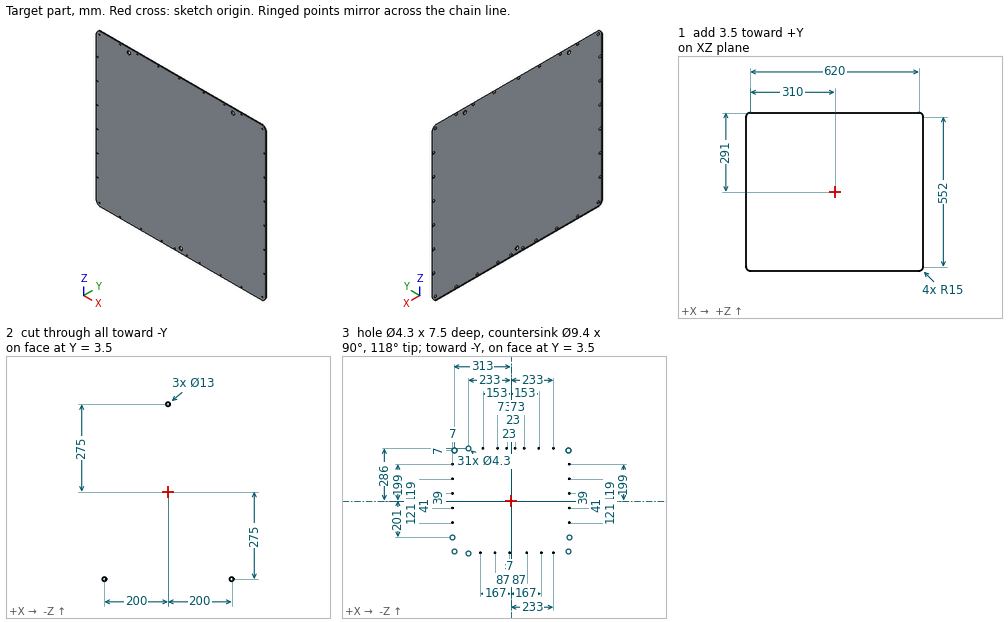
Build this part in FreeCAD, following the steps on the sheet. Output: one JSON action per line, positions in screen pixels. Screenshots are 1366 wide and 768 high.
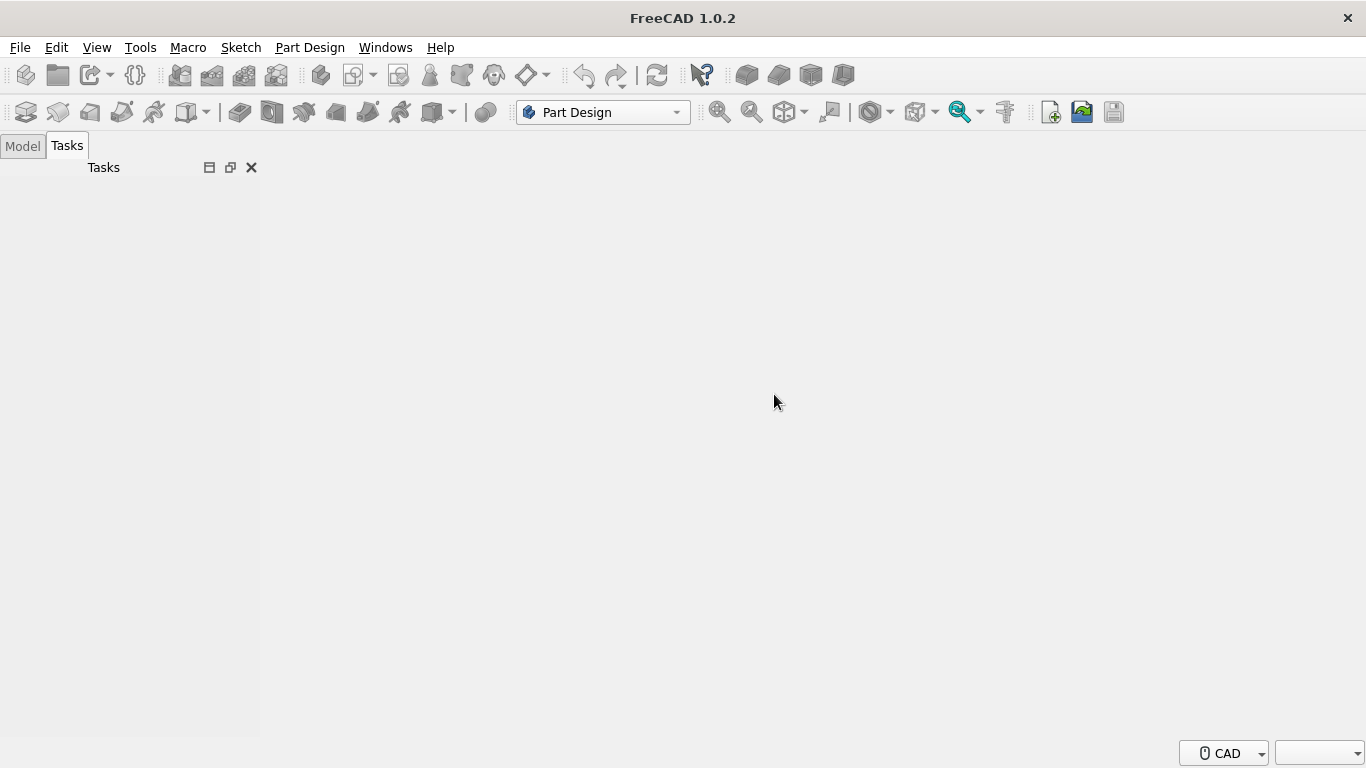
{"action": "left_click", "coordinate": [1050, 112]}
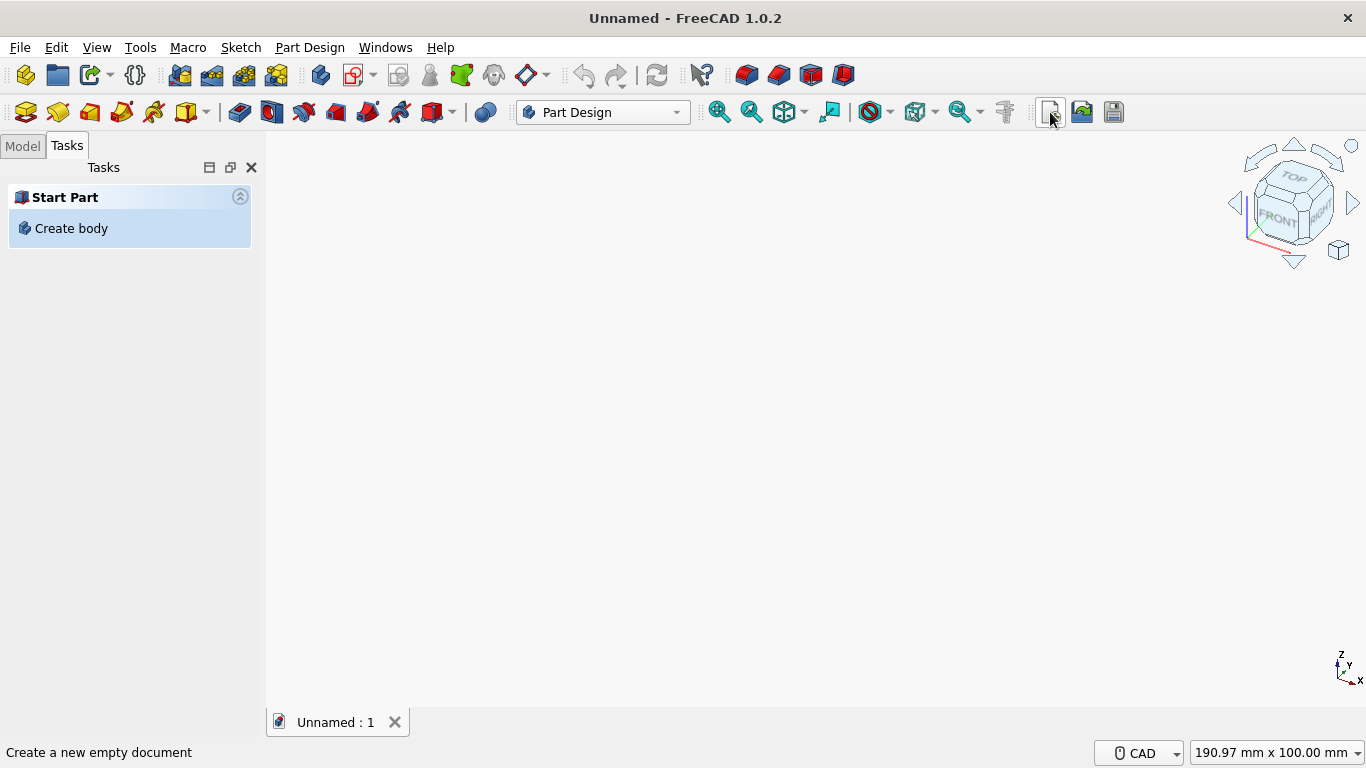
{"action": "left_click", "coordinate": [354, 76]}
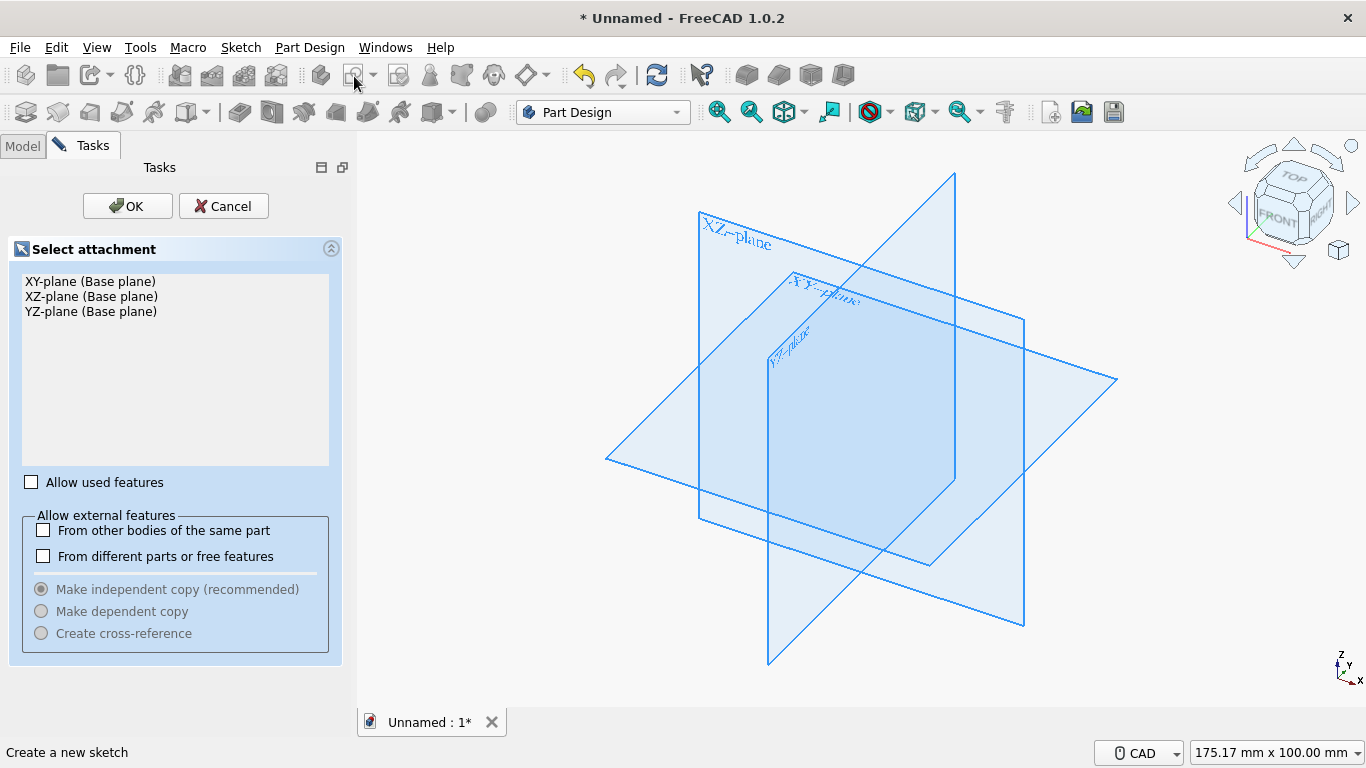
{"action": "left_click", "coordinate": [82, 296]}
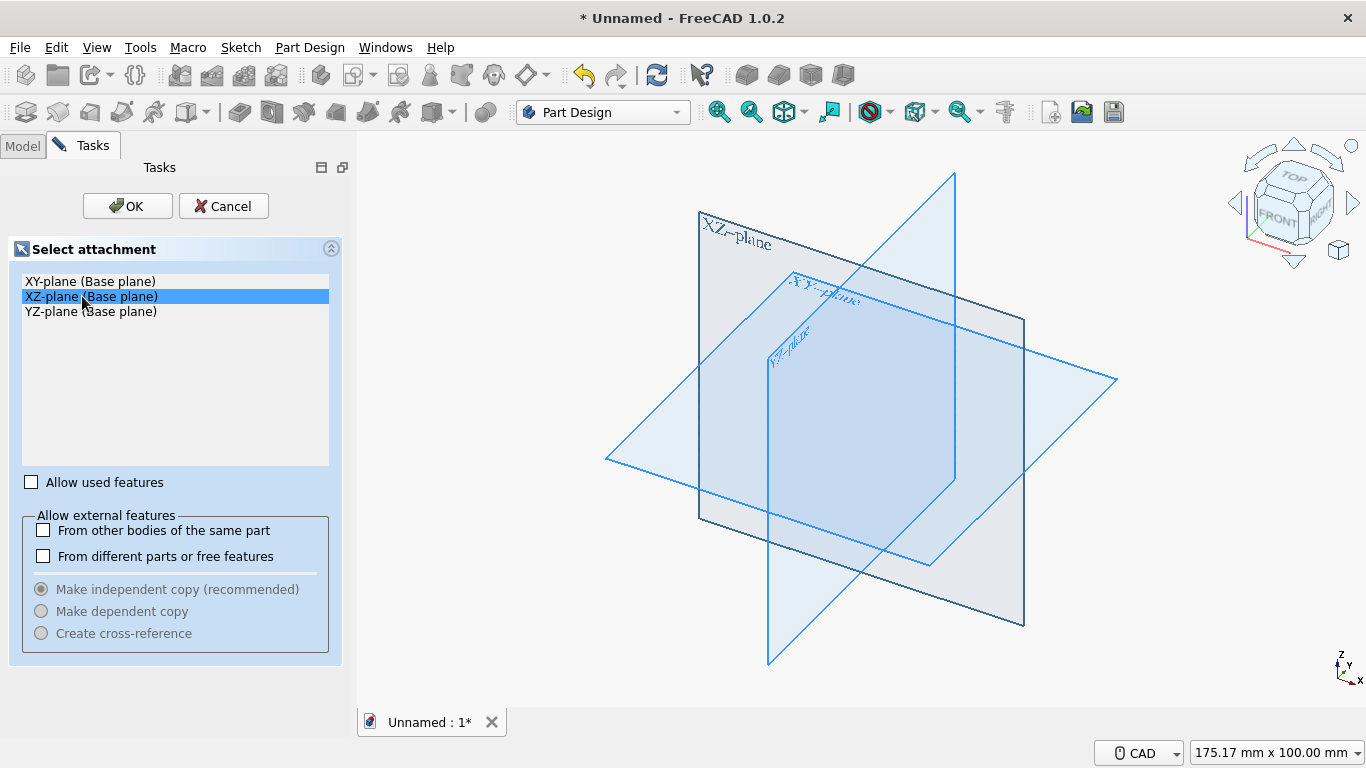
{"action": "left_click", "coordinate": [128, 206]}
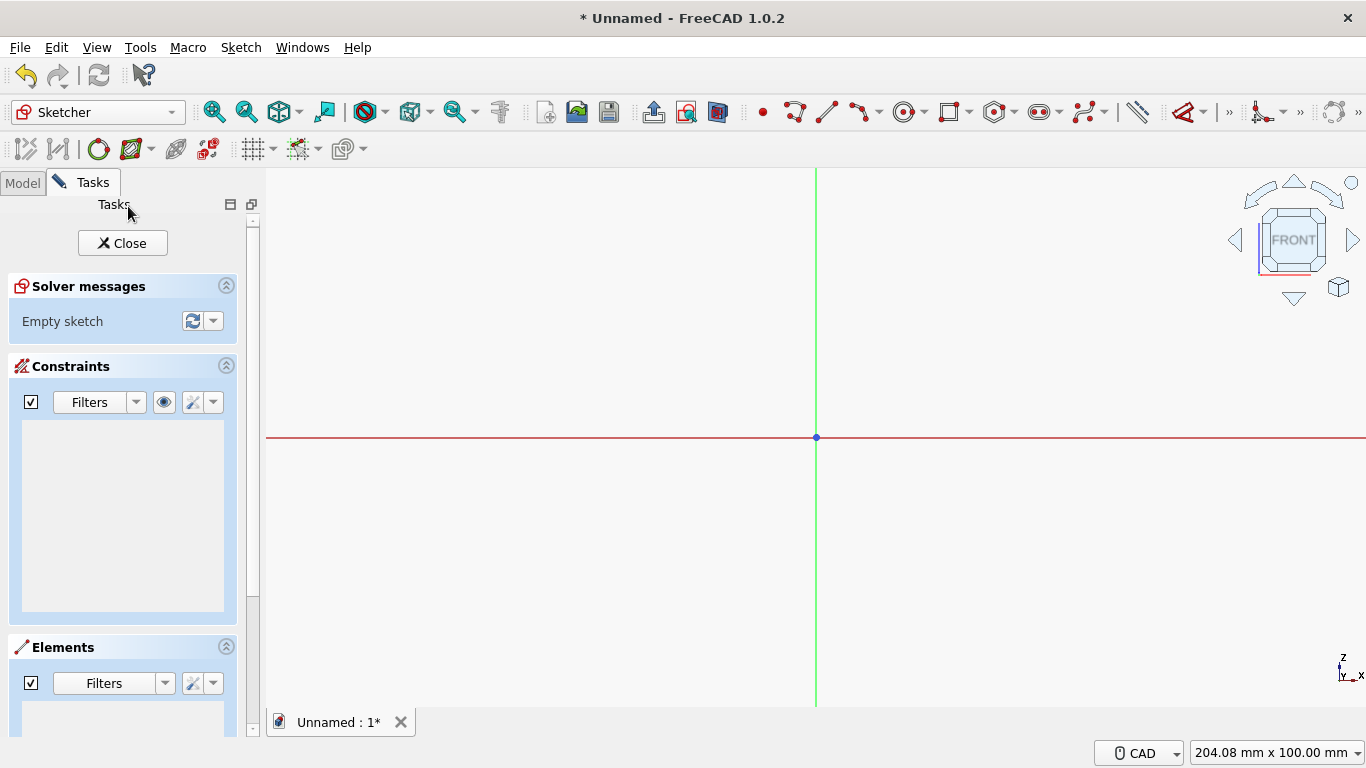
{"action": "scroll", "coordinate": [739, 438], "scroll_direction": "down", "scroll_amount": 11}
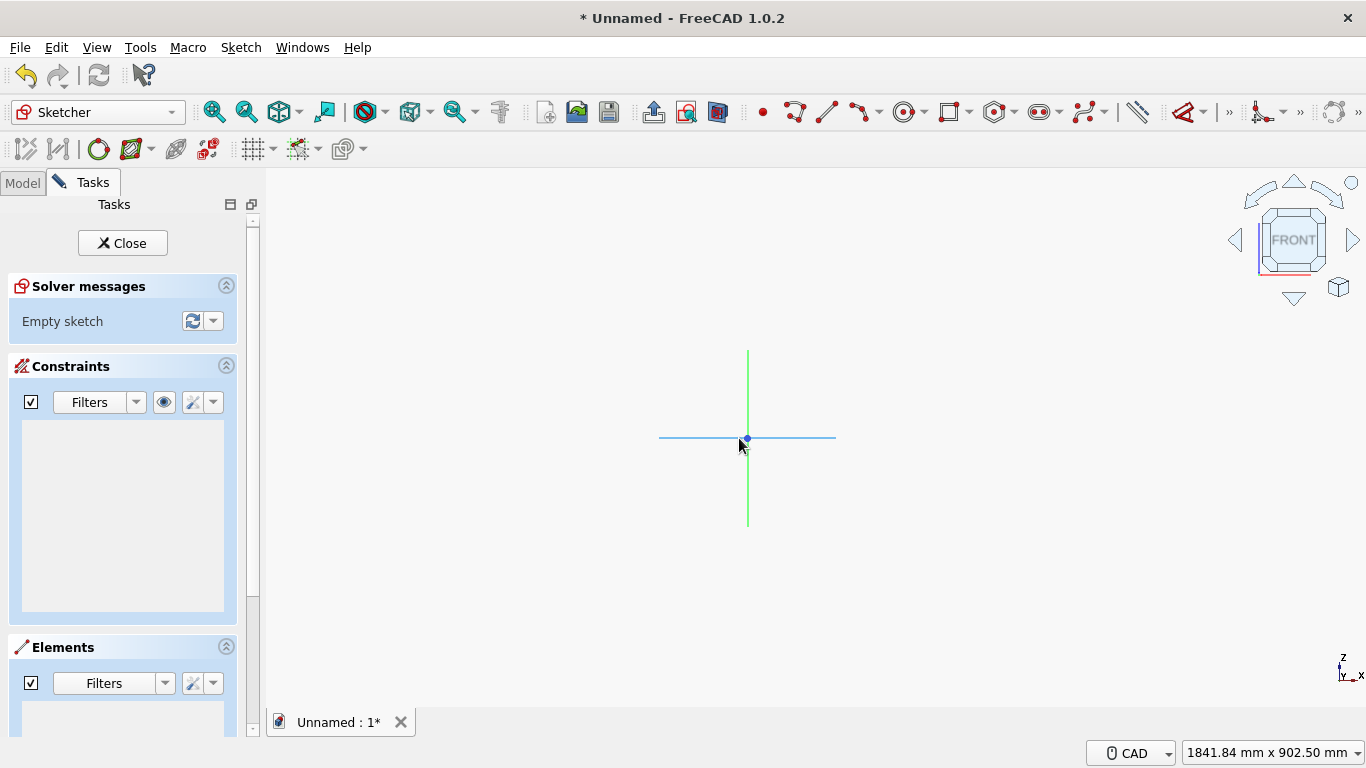
{"action": "left_click", "coordinate": [828, 112]}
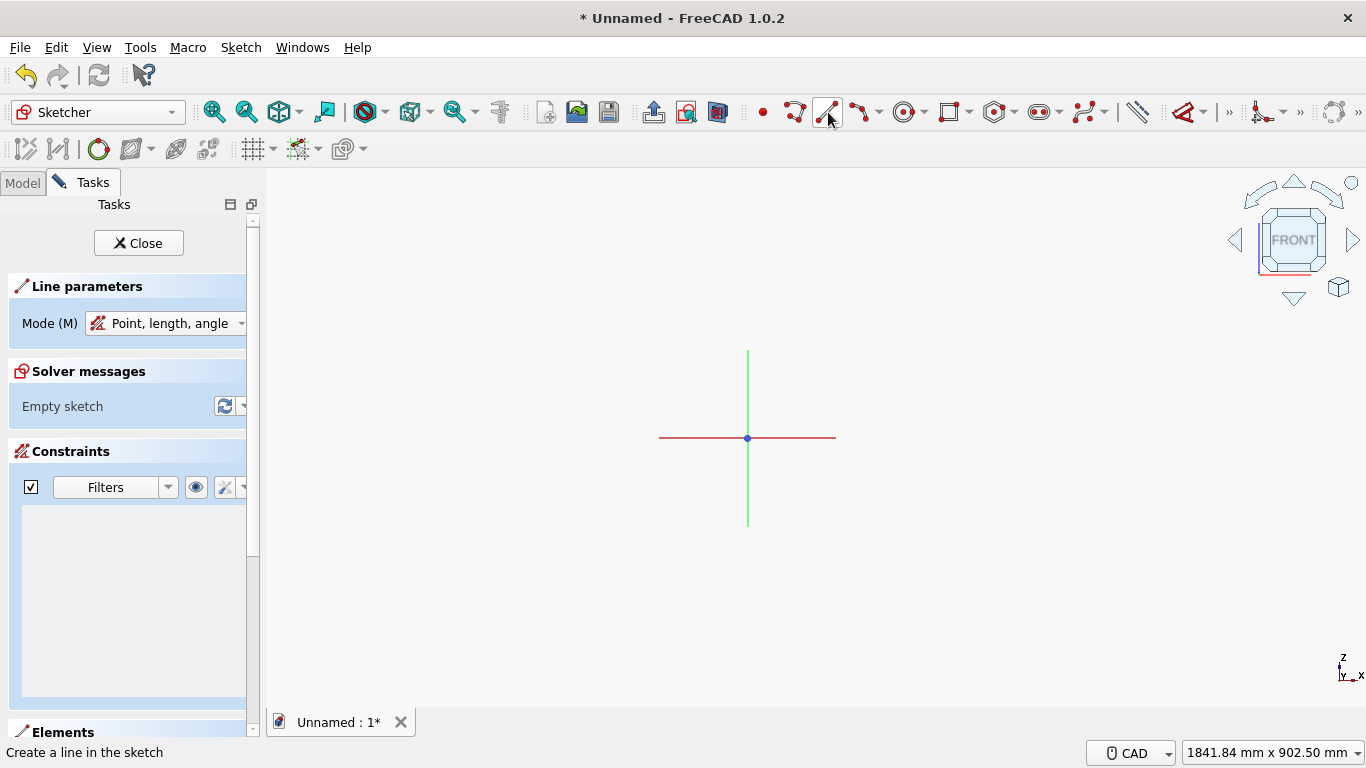
{"action": "left_click", "coordinate": [563, 265]}
{"action": "left_click", "coordinate": [933, 265]}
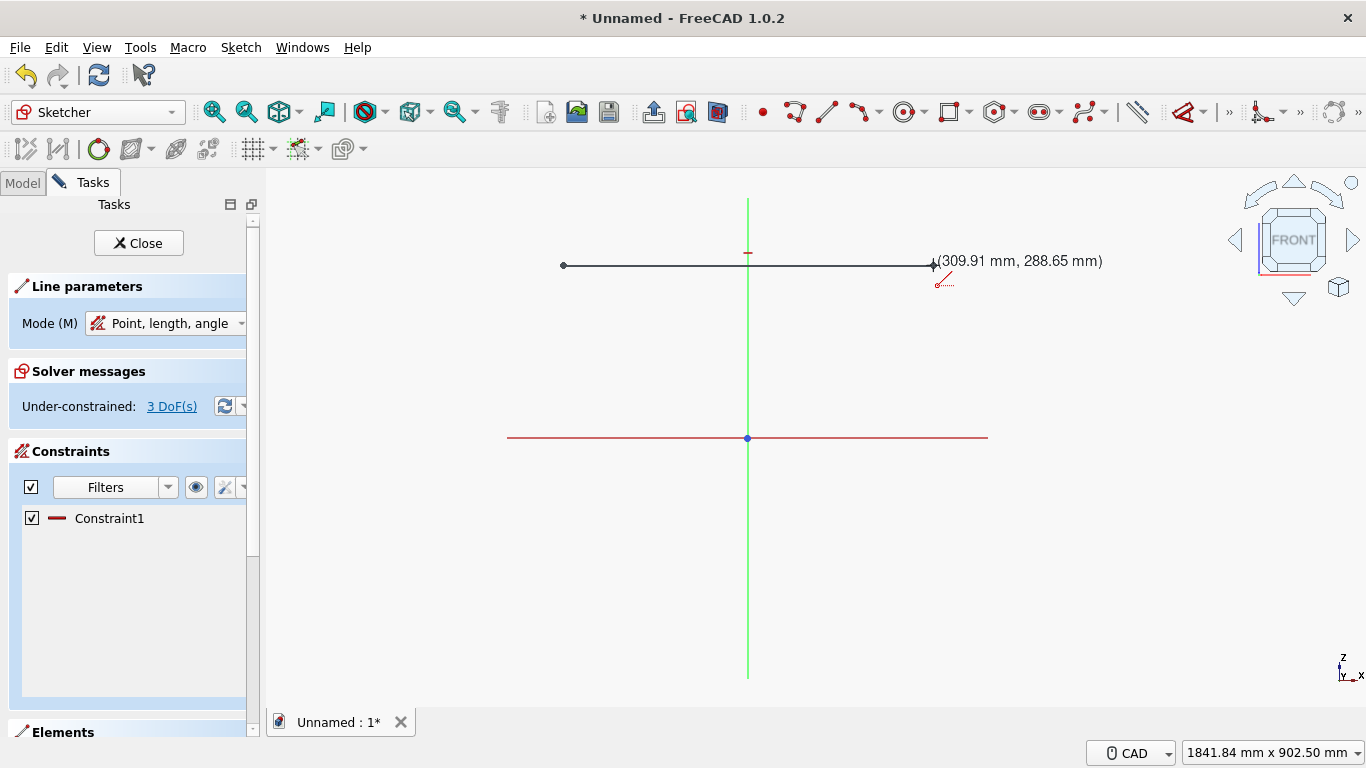
{"action": "scroll", "coordinate": [942, 274], "scroll_direction": "up", "scroll_amount": 2}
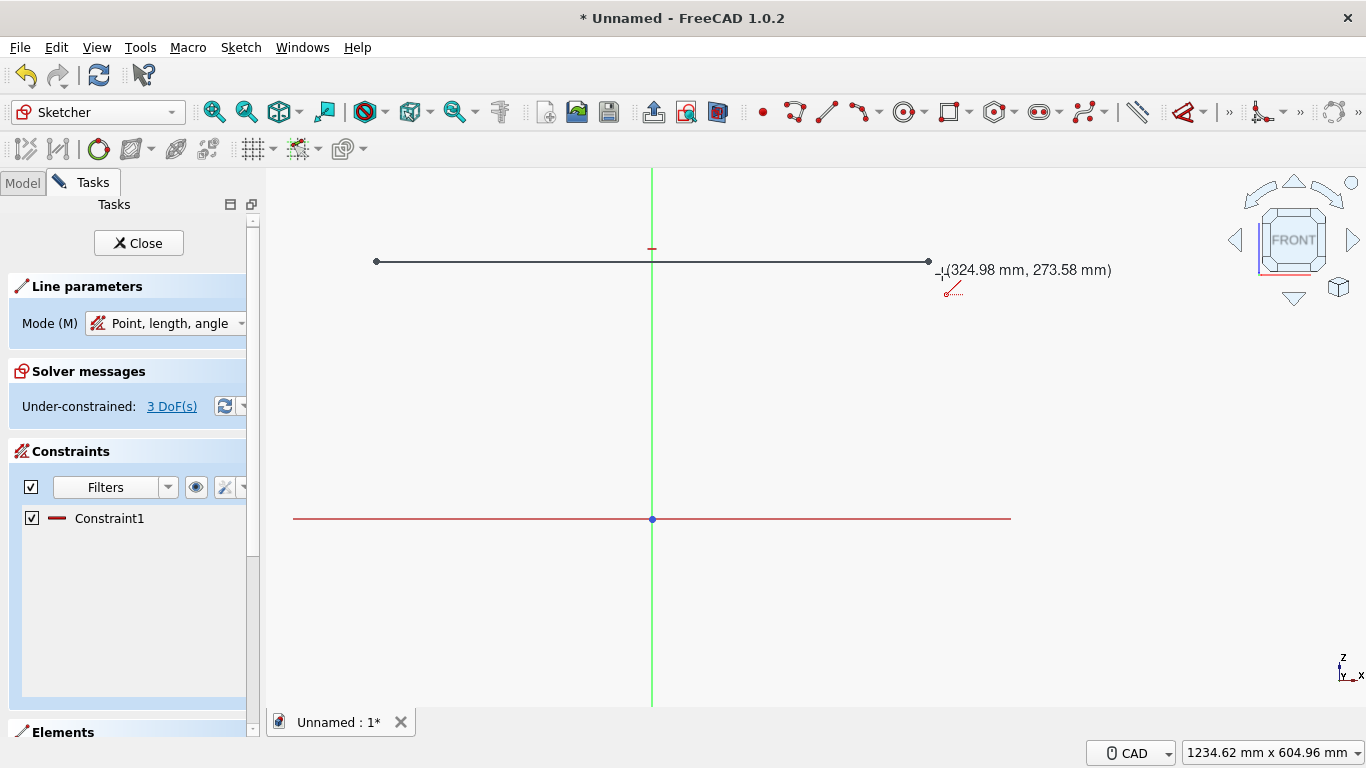
{"action": "left_click", "coordinate": [942, 273]}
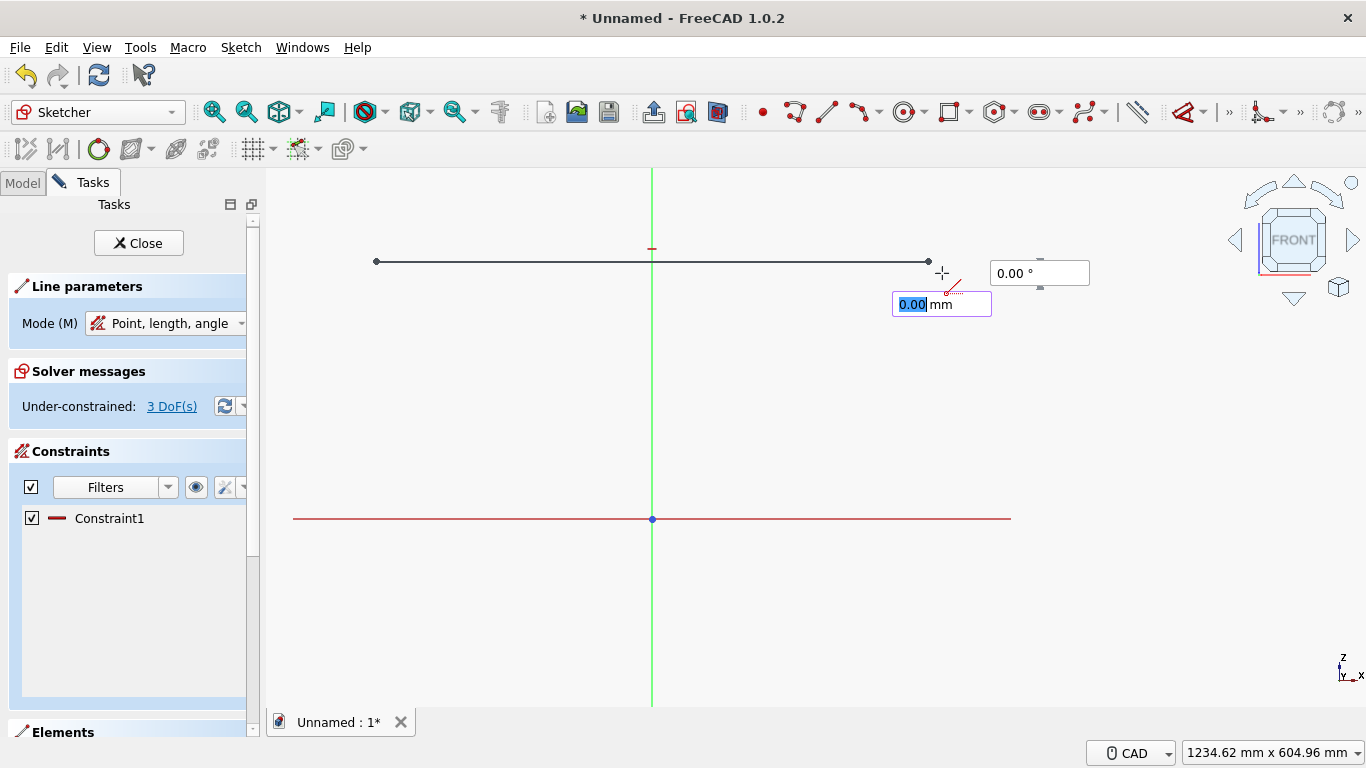
{"action": "scroll", "coordinate": [941, 271], "scroll_direction": "down", "scroll_amount": 2}